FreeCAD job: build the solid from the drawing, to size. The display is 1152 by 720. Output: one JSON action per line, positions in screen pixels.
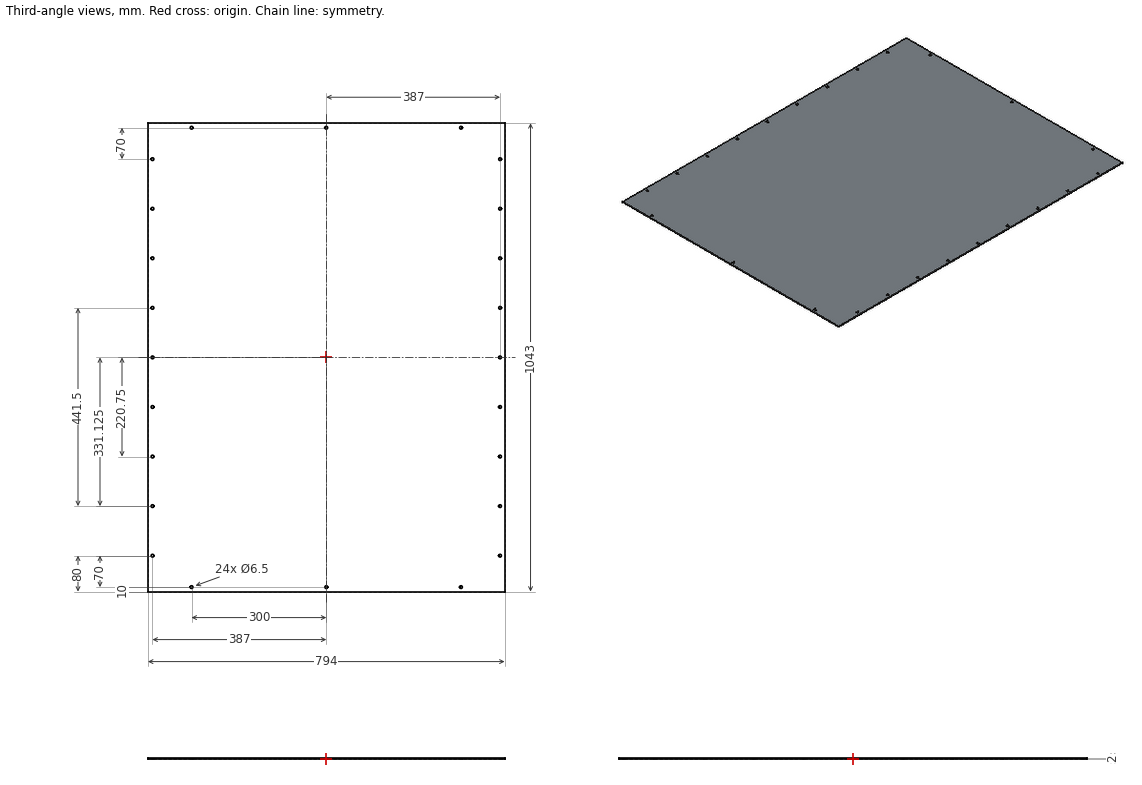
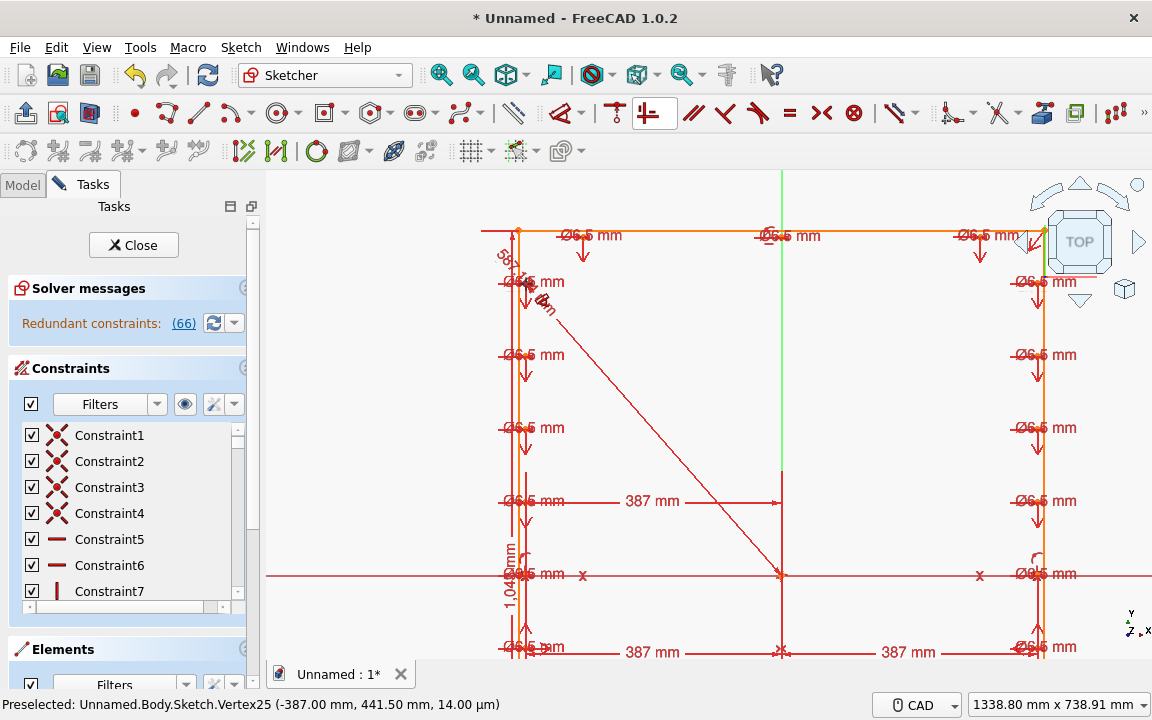
{"action": "left_click", "coordinate": [782, 238]}
{"action": "left_click", "coordinate": [492, 261]}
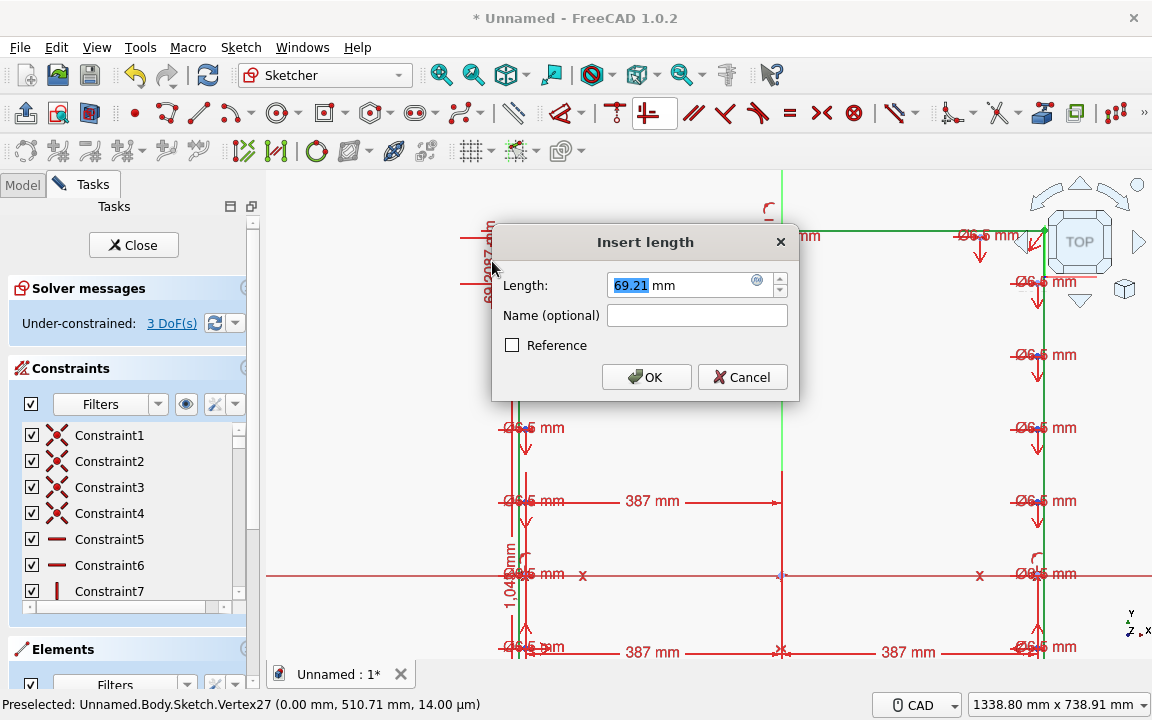
{"action": "type", "text": "70"}
{"action": "key", "text": "Return"}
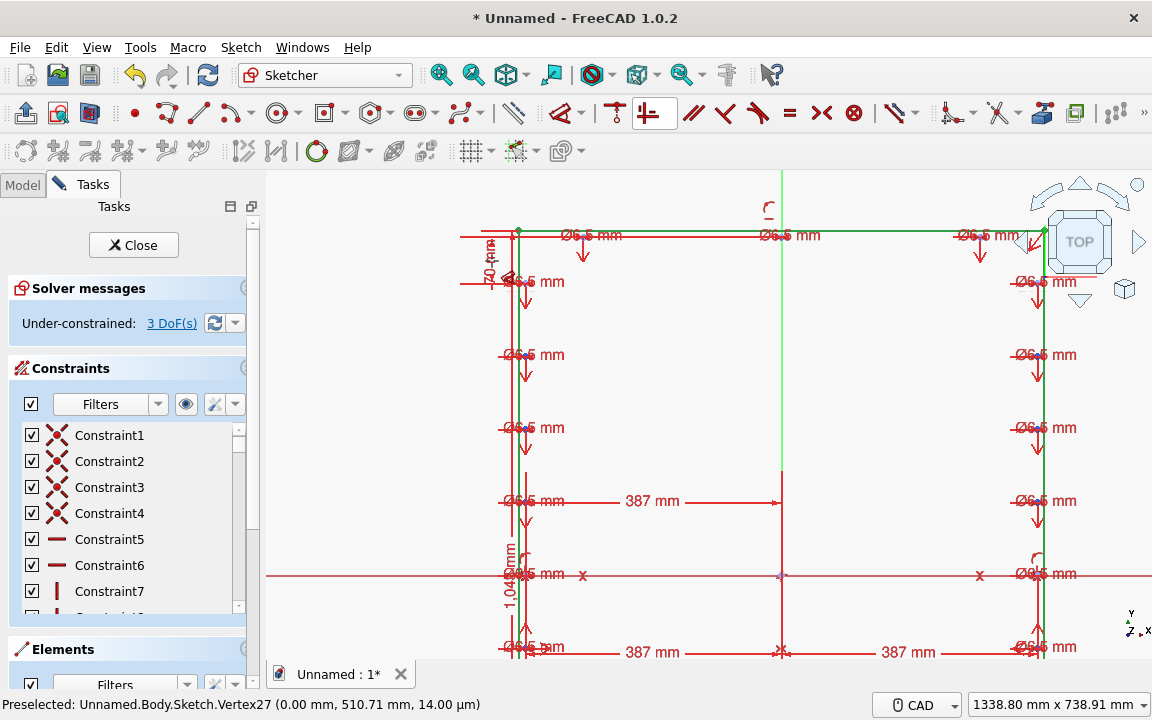
{"action": "scroll", "coordinate": [525, 283], "scroll_direction": "down", "scroll_amount": 4}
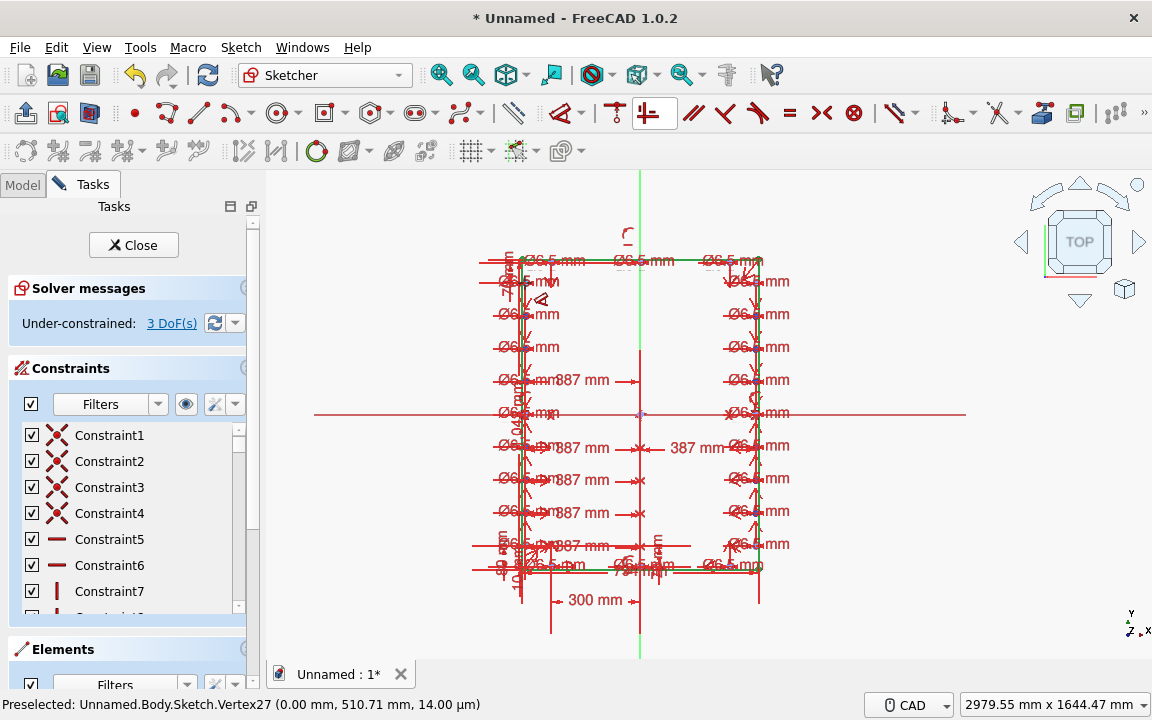
{"action": "left_click", "coordinate": [525, 480]}
{"action": "left_click", "coordinate": [491, 448]}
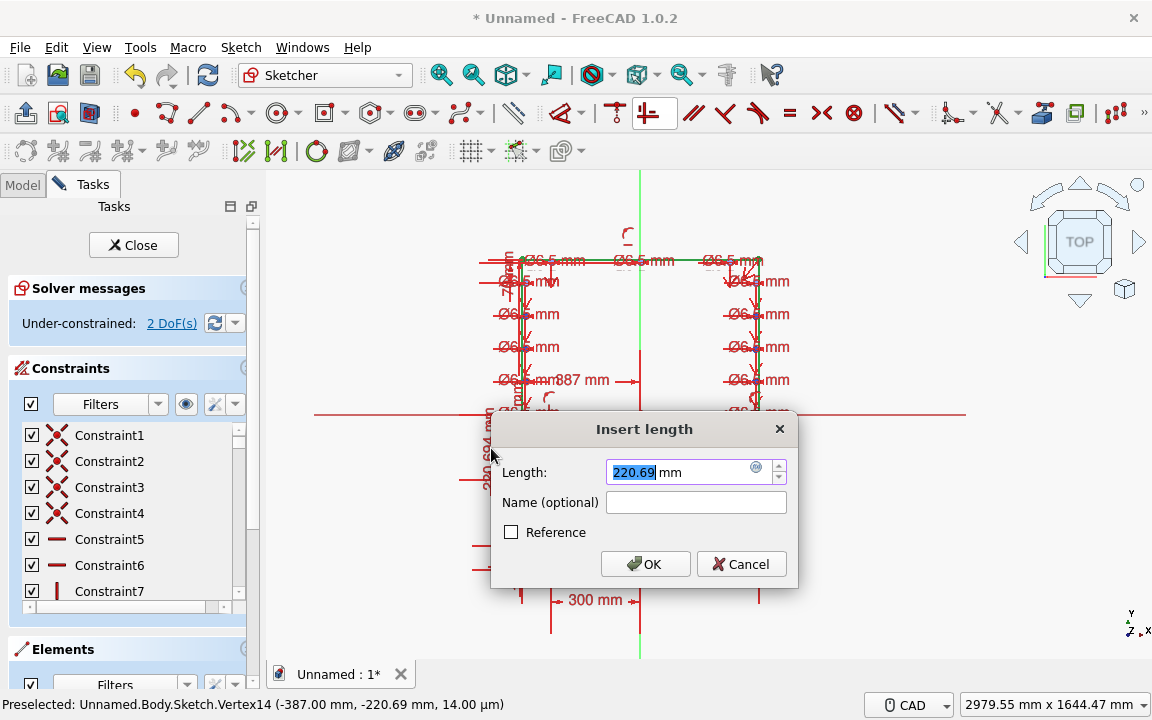
{"action": "type", "text": "220.75"}
{"action": "key", "text": "Return"}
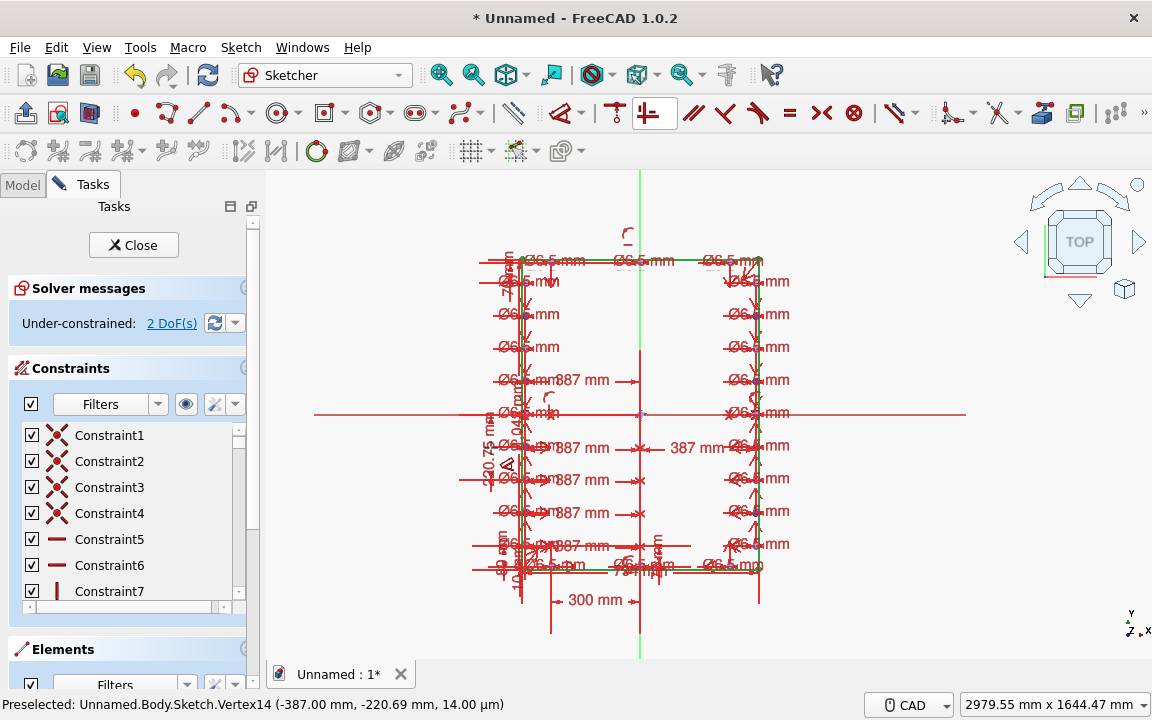
{"action": "left_click", "coordinate": [525, 513]}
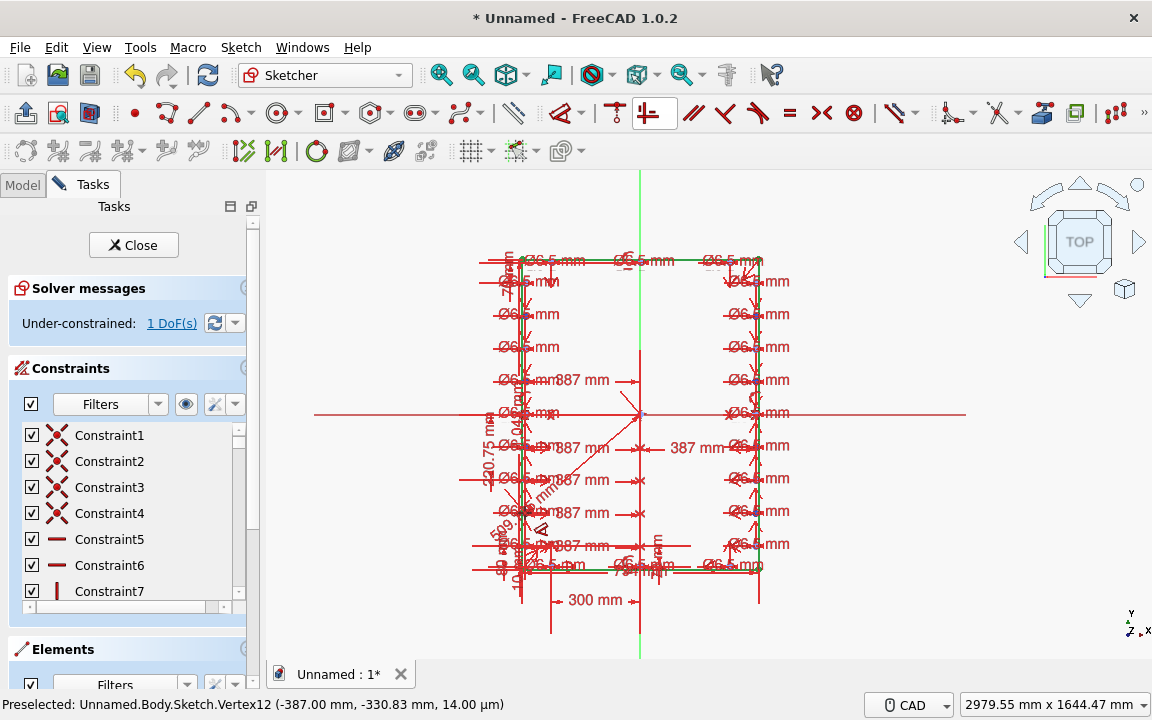
{"action": "left_click", "coordinate": [525, 382]}
{"action": "left_click", "coordinate": [491, 478]}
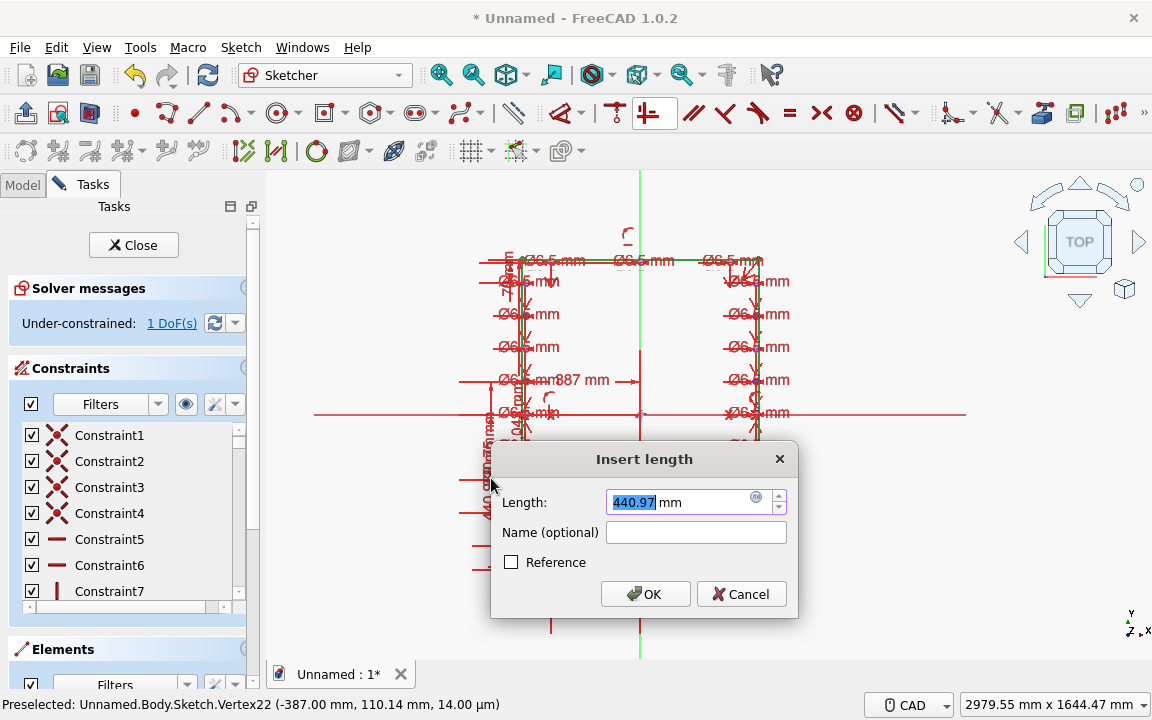
{"action": "type", "text": "441.5"}
{"action": "key", "text": "Return"}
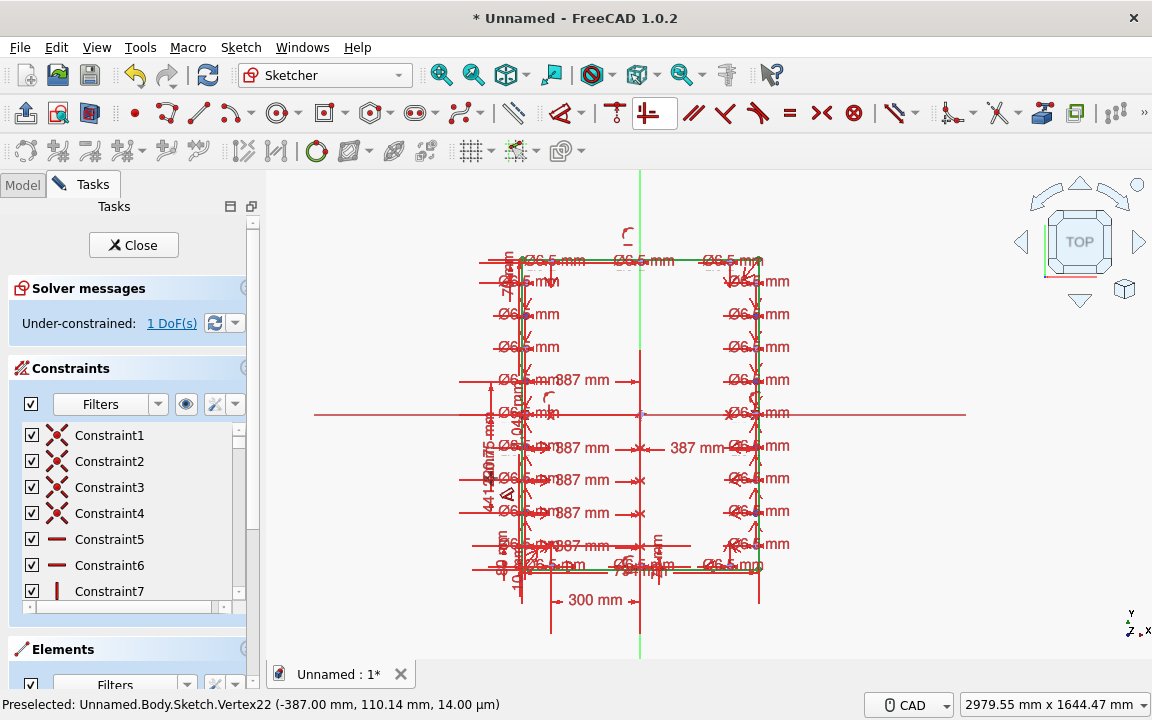
{"action": "left_click", "coordinate": [525, 513]}
{"action": "left_click", "coordinate": [491, 498]}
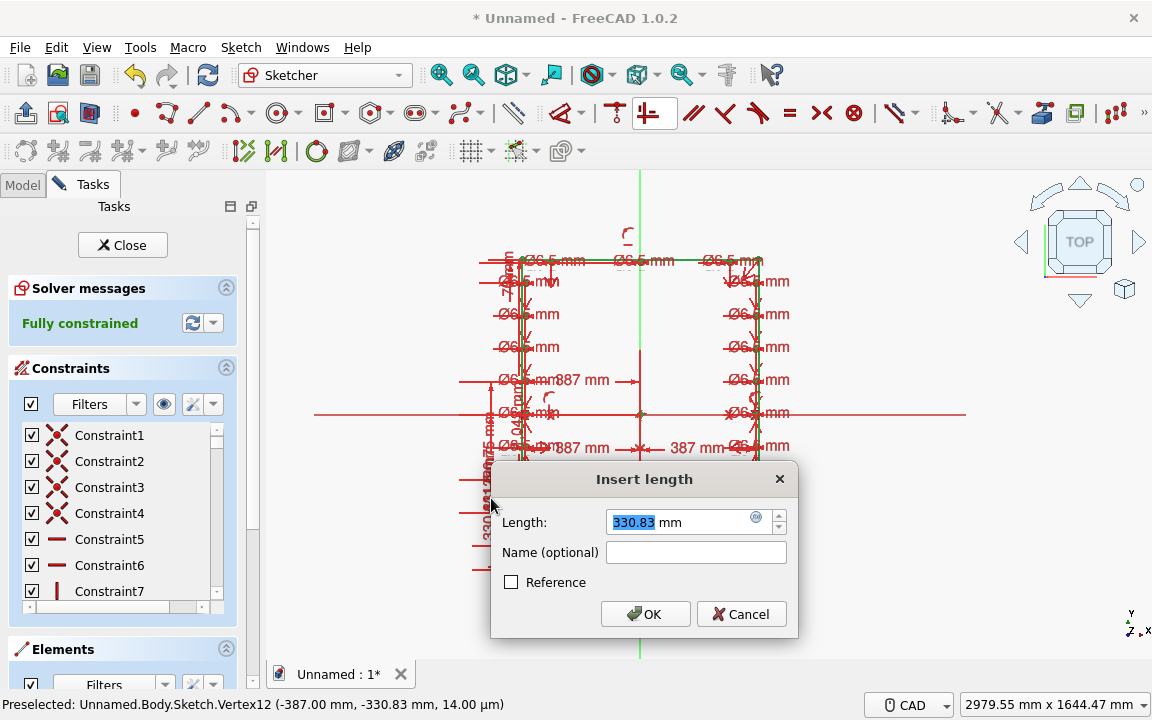
{"action": "type", "text": "331.125"}
{"action": "key", "text": "Return"}
{"action": "key", "text": "Escape"}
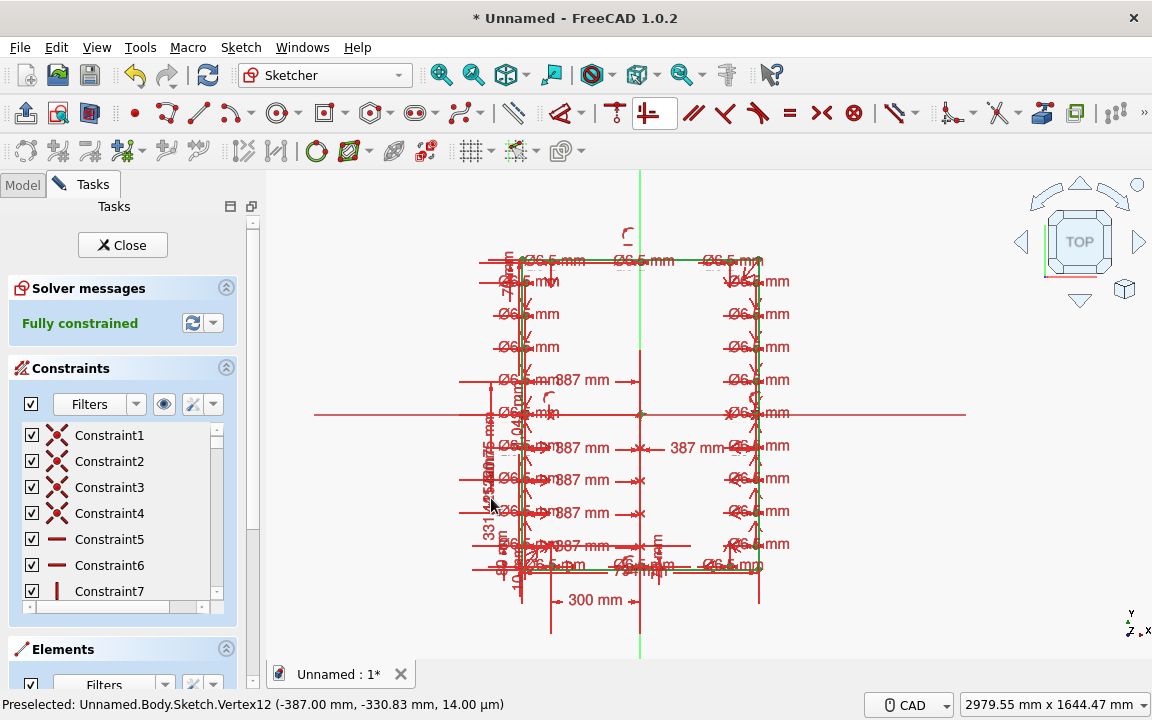
{"action": "left_click", "coordinate": [123, 245]}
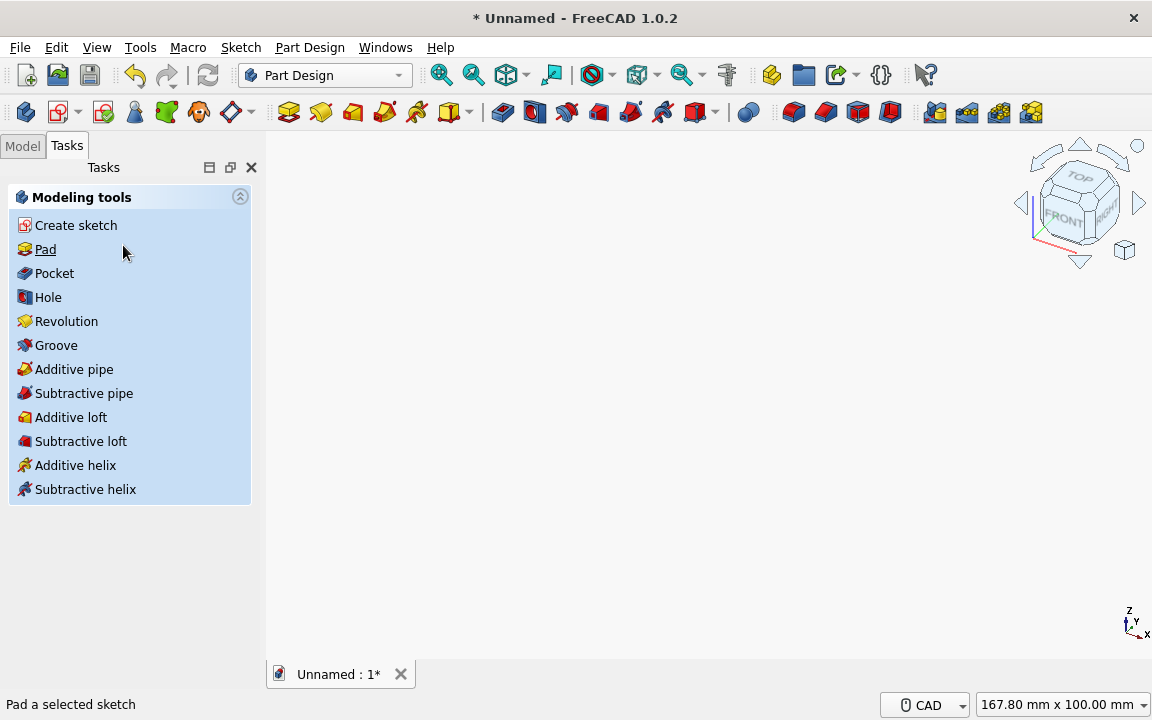
{"action": "left_click", "coordinate": [290, 112]}